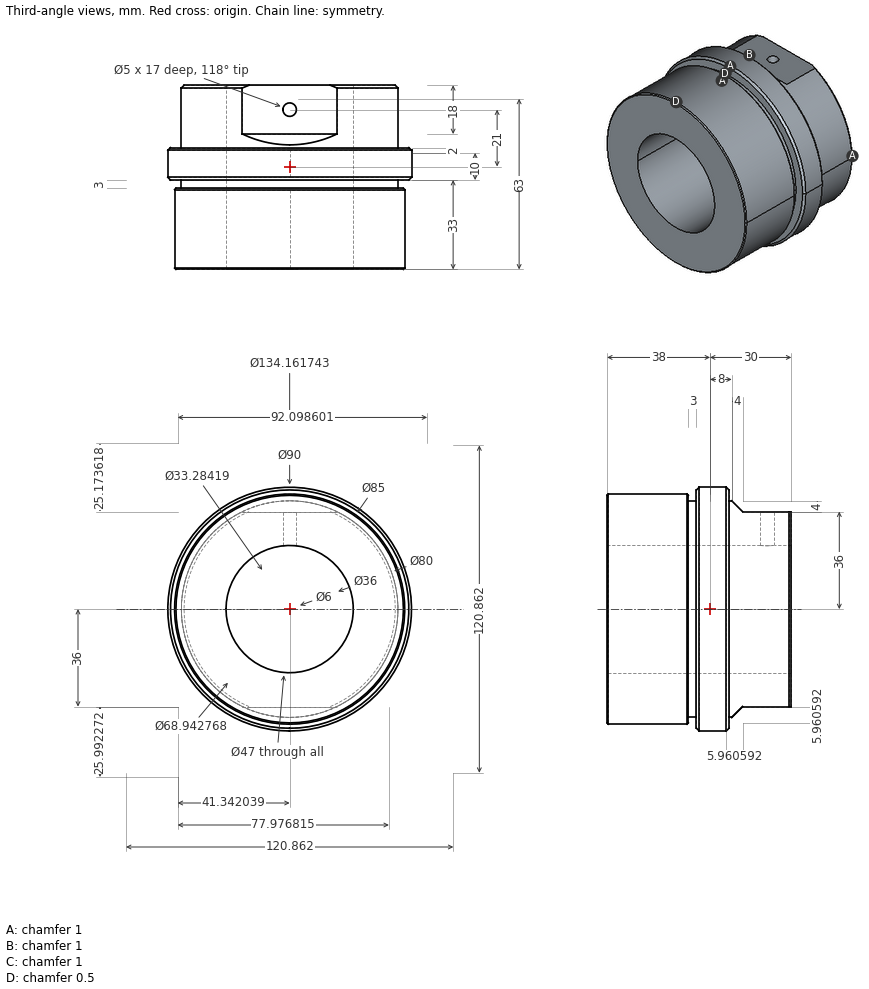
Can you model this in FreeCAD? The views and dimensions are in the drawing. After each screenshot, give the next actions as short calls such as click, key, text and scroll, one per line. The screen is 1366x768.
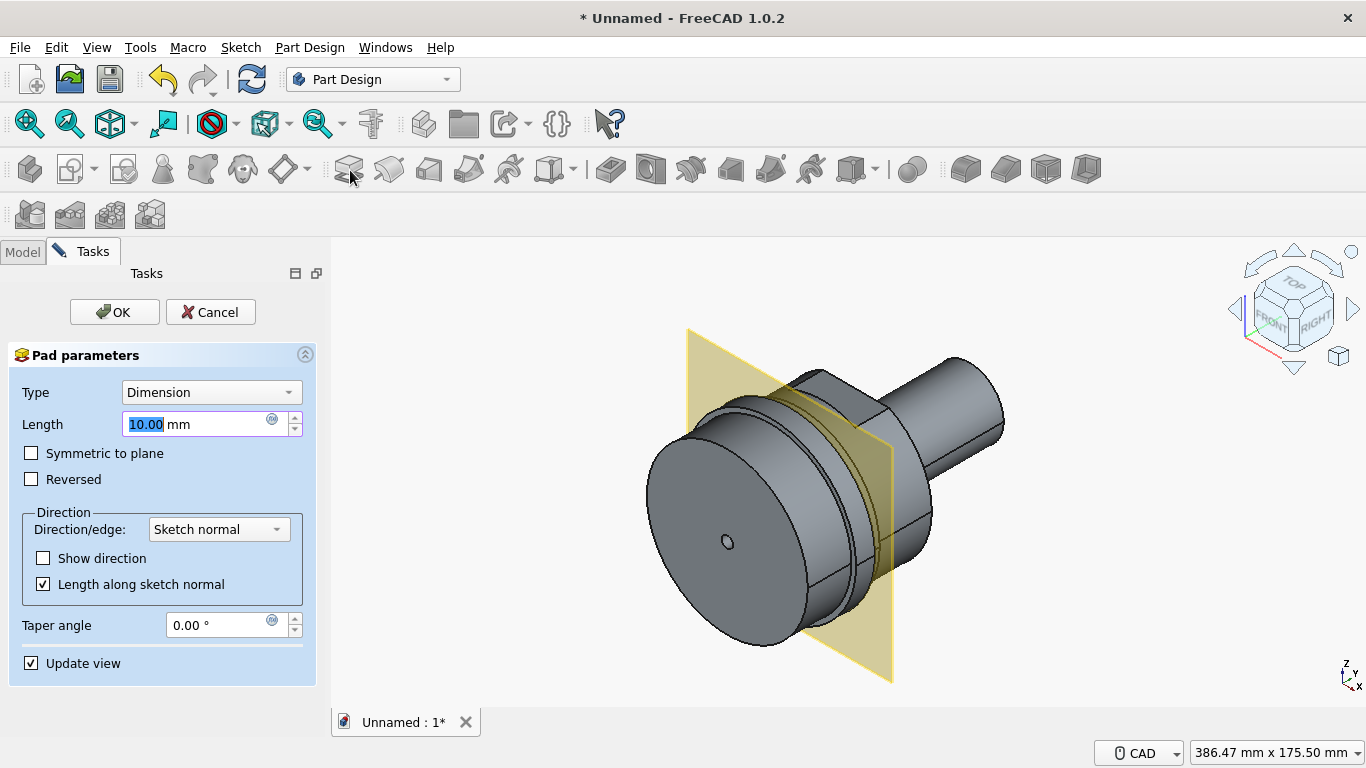
text(10)
key(Tab)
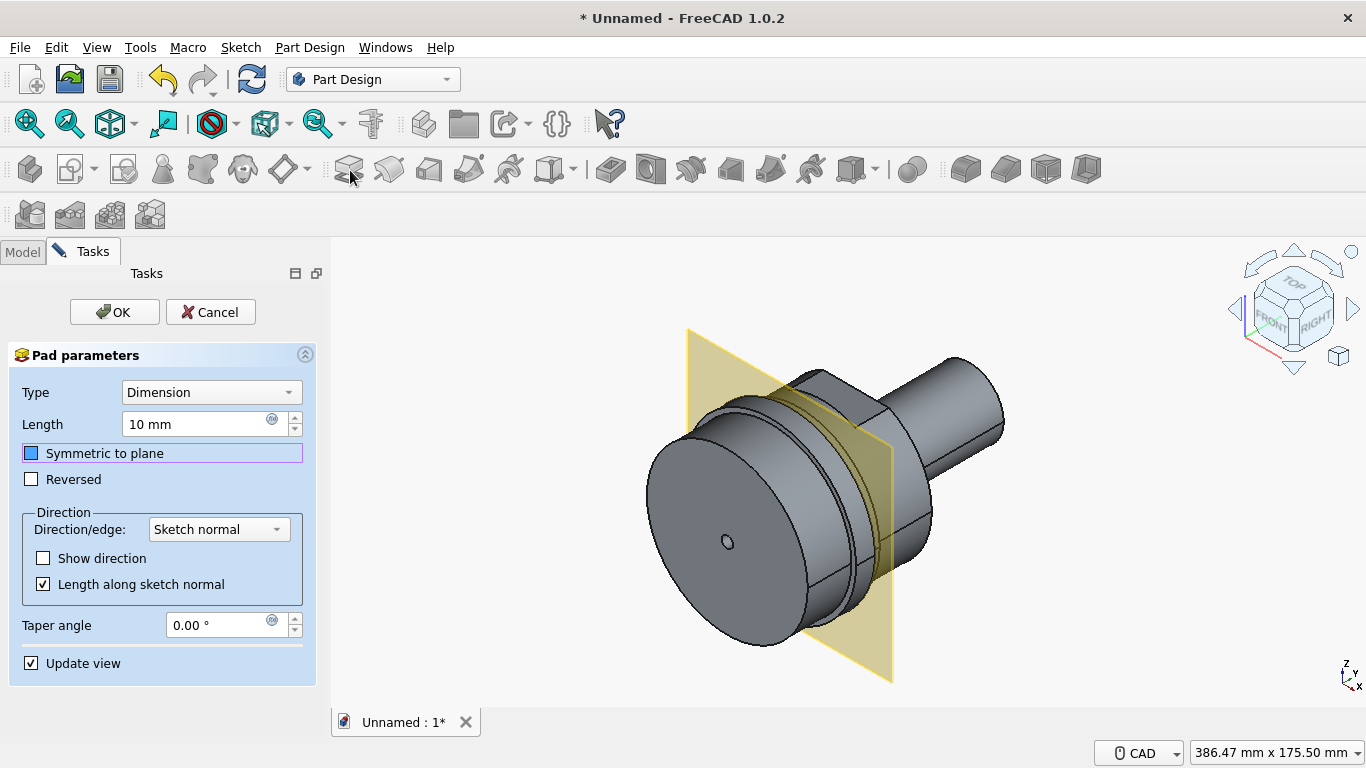
click(30, 479)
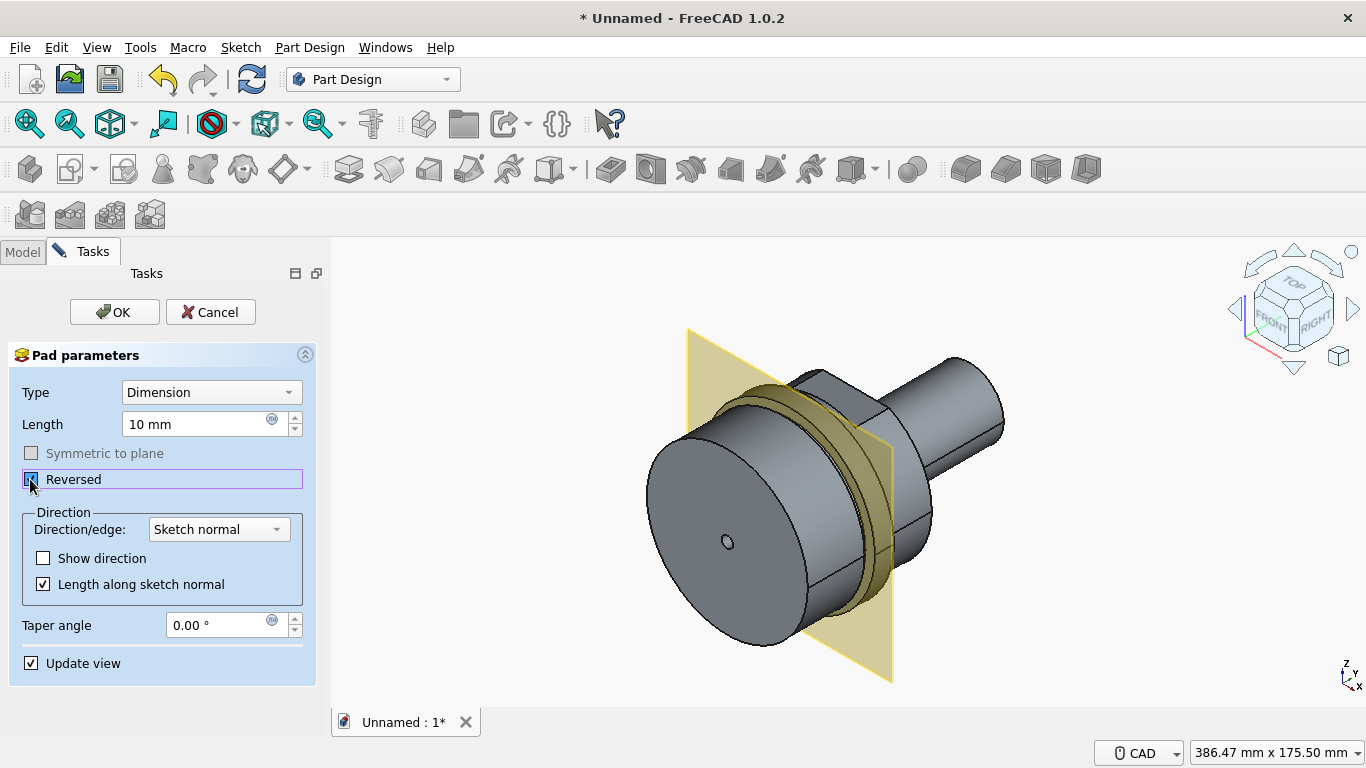
click(115, 312)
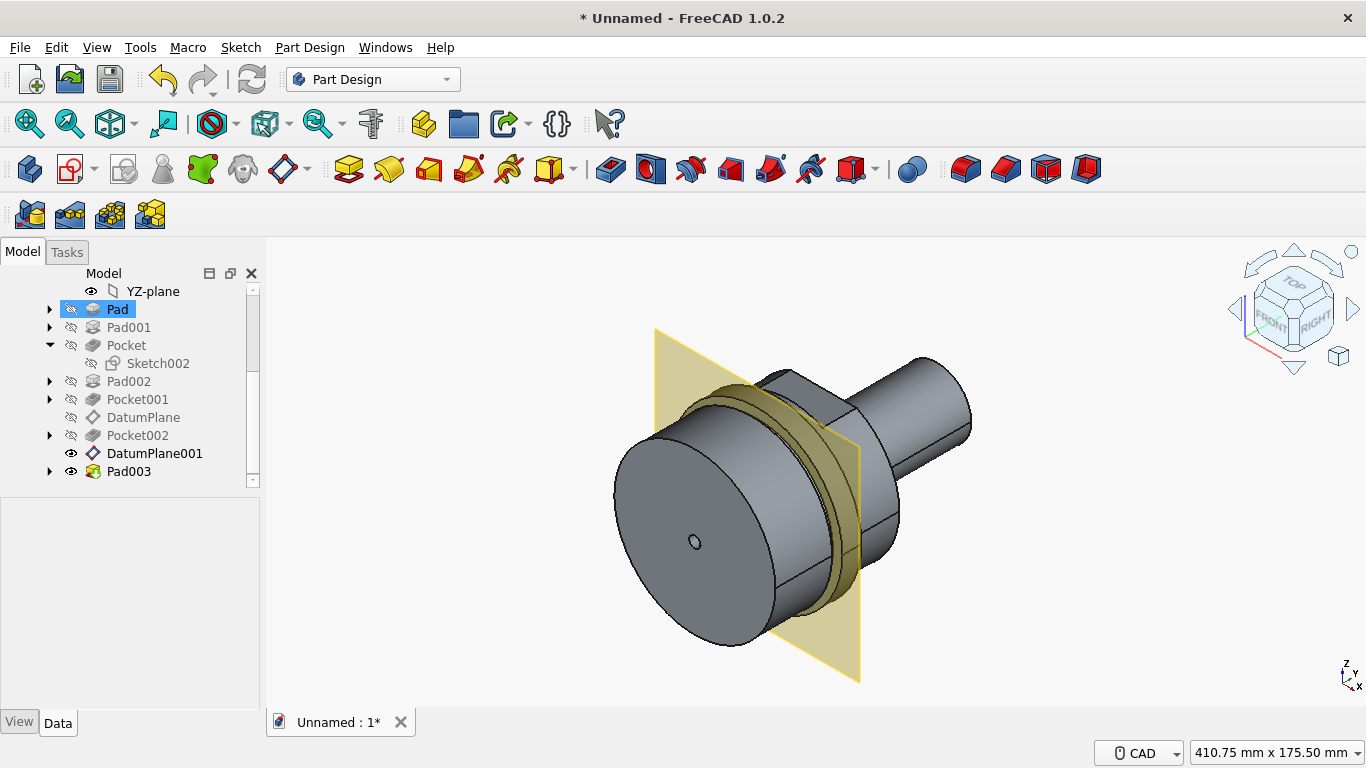
click(116, 453)
key(space)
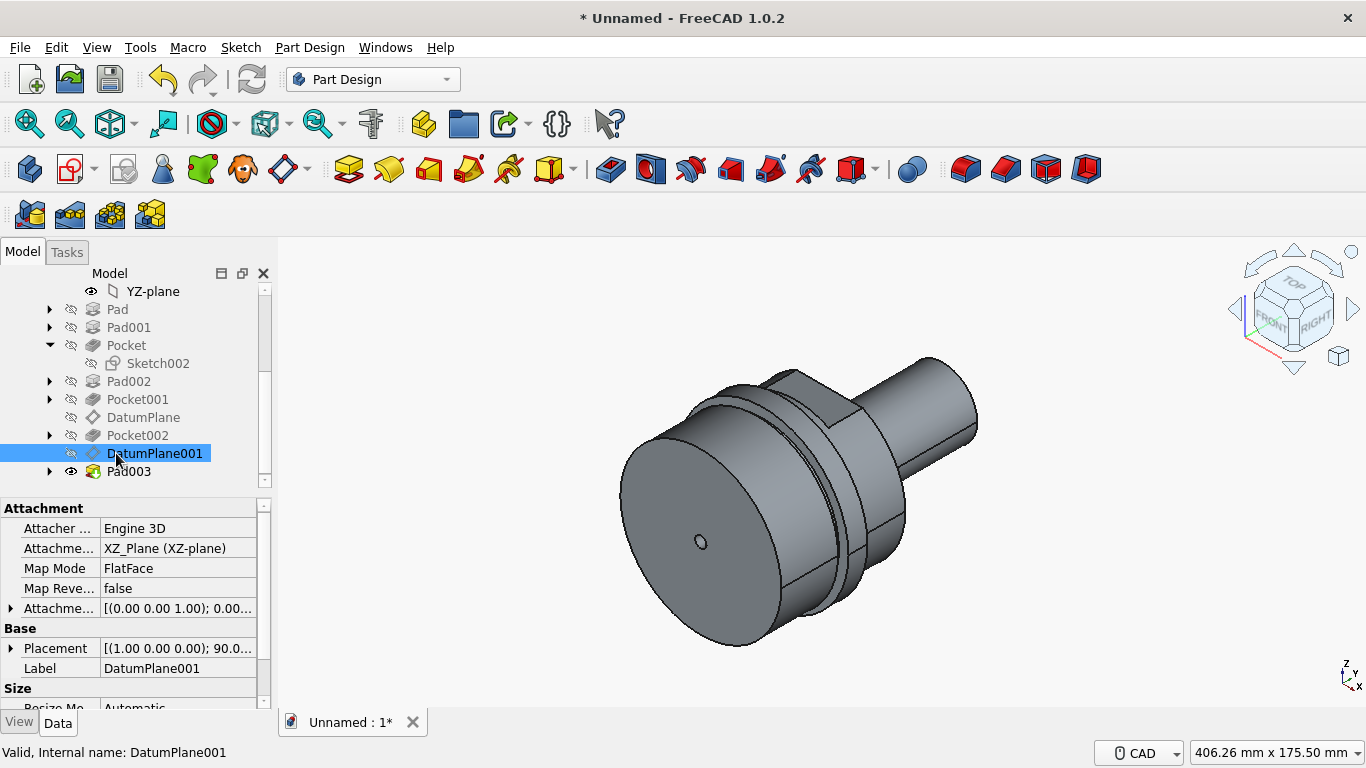
click(676, 438)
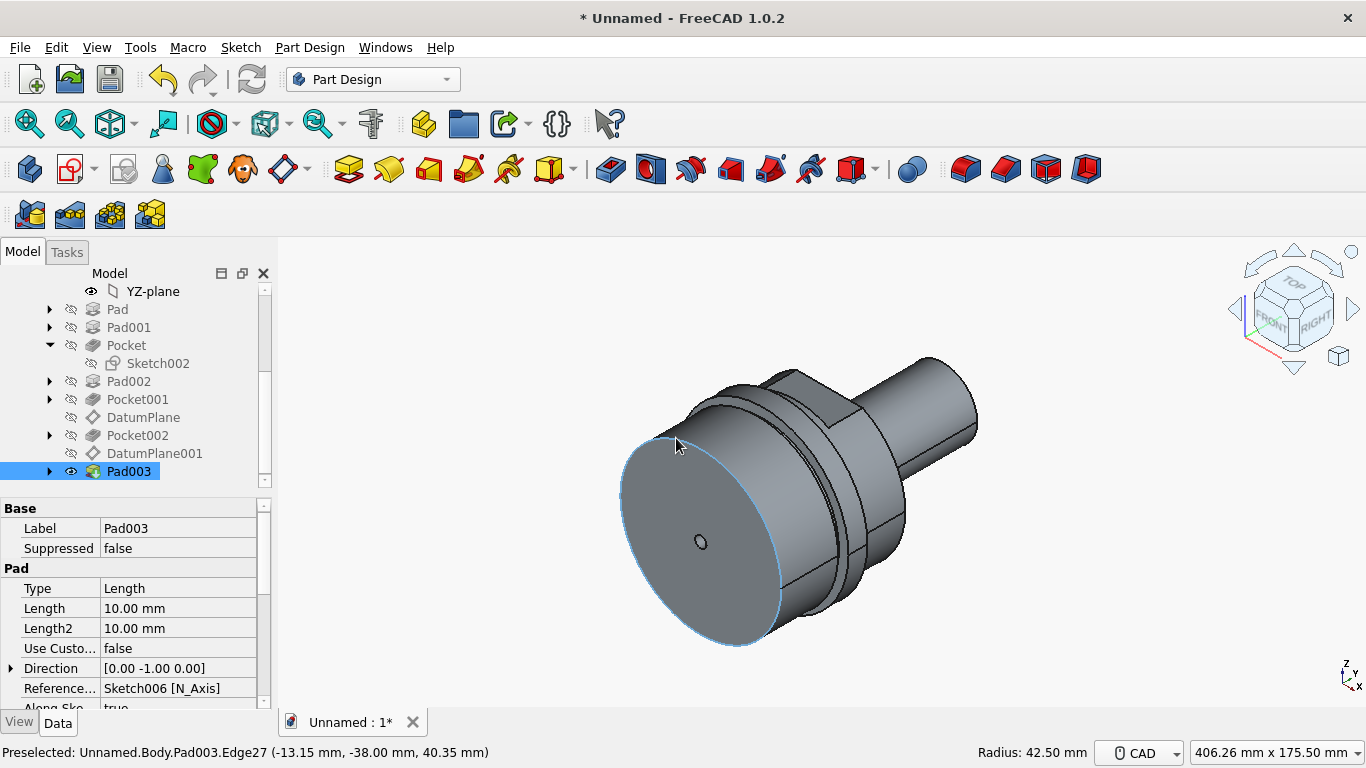
click(737, 396, ctrl)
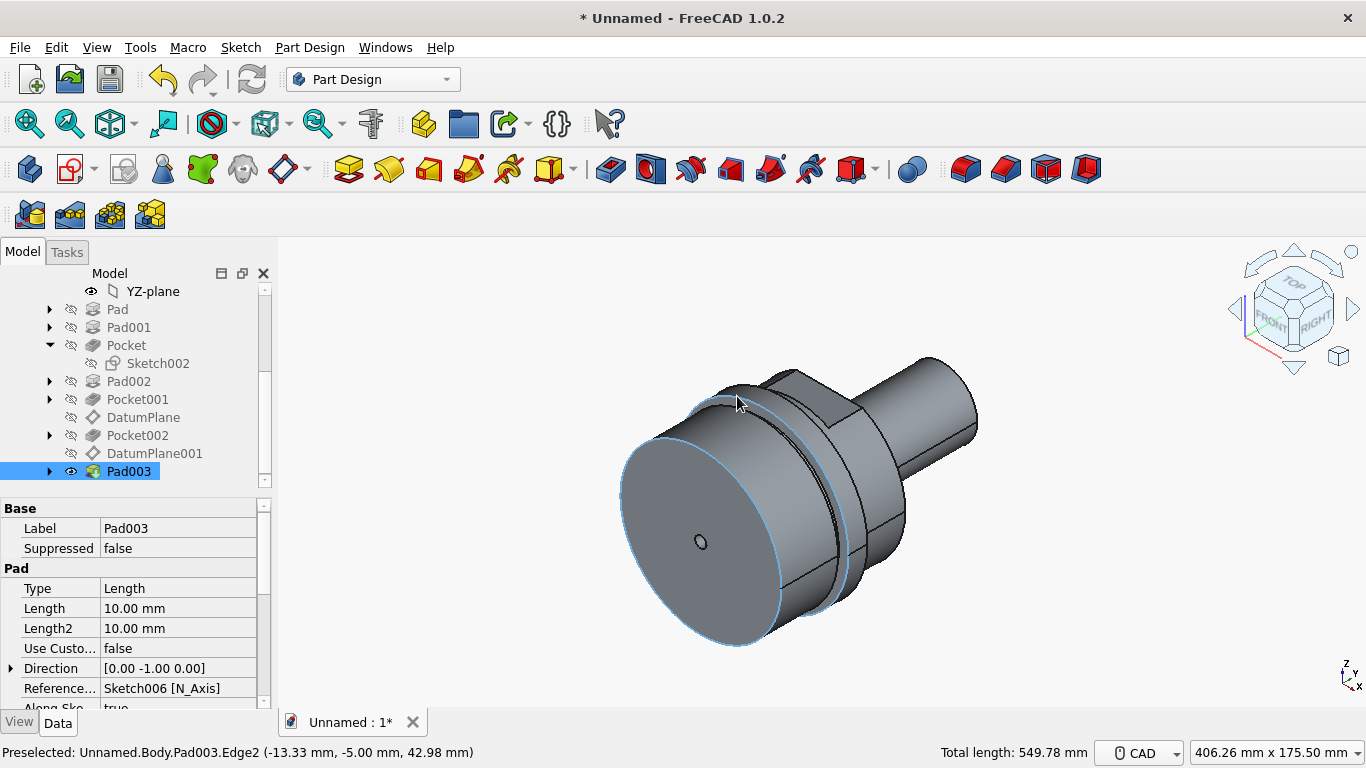
key(2)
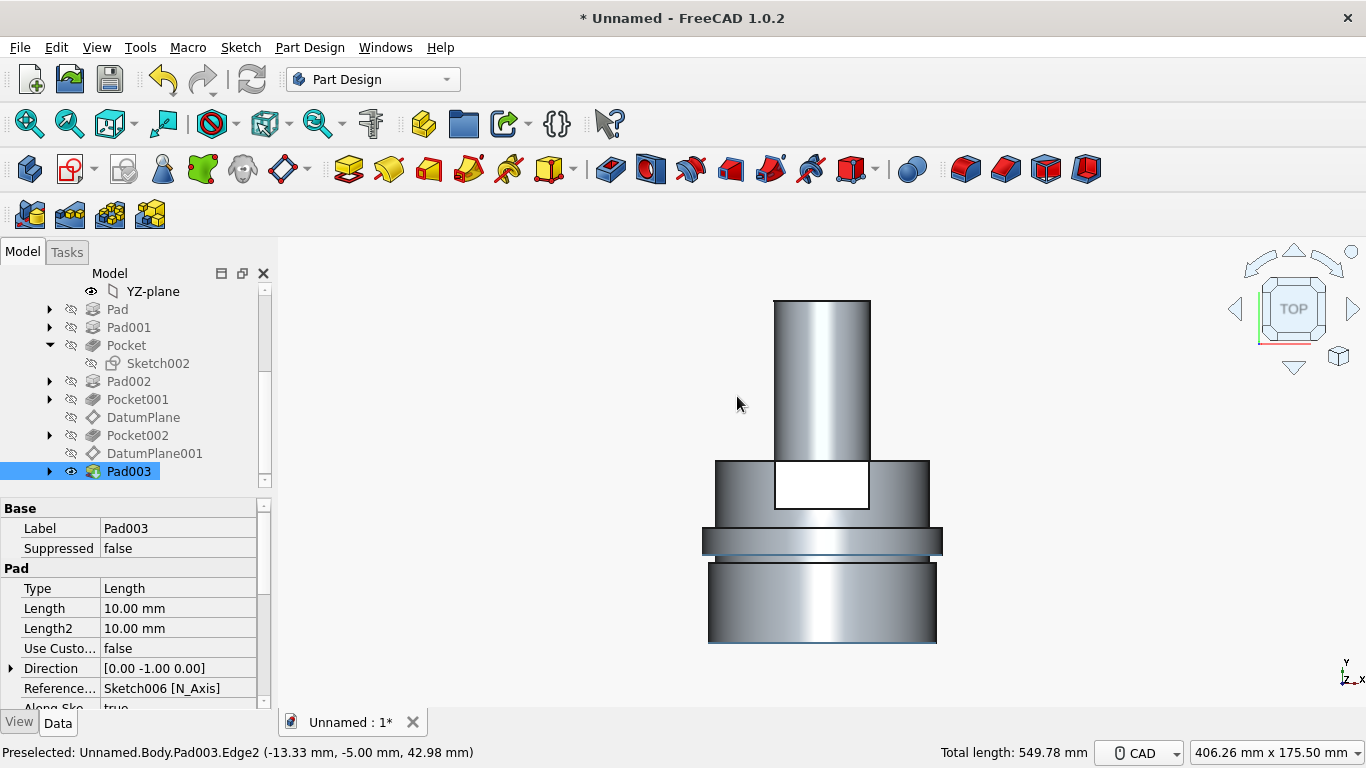
click(783, 300, ctrl)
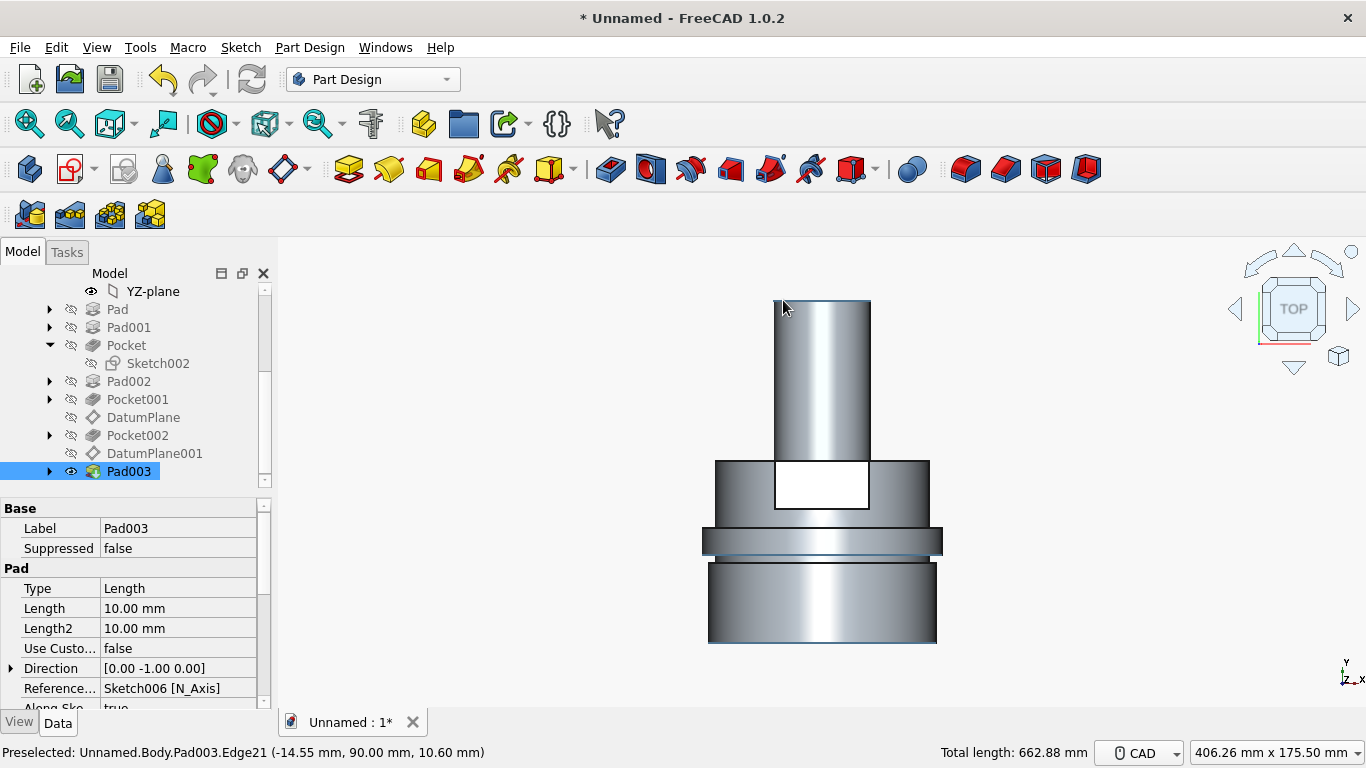
click(738, 460, ctrl)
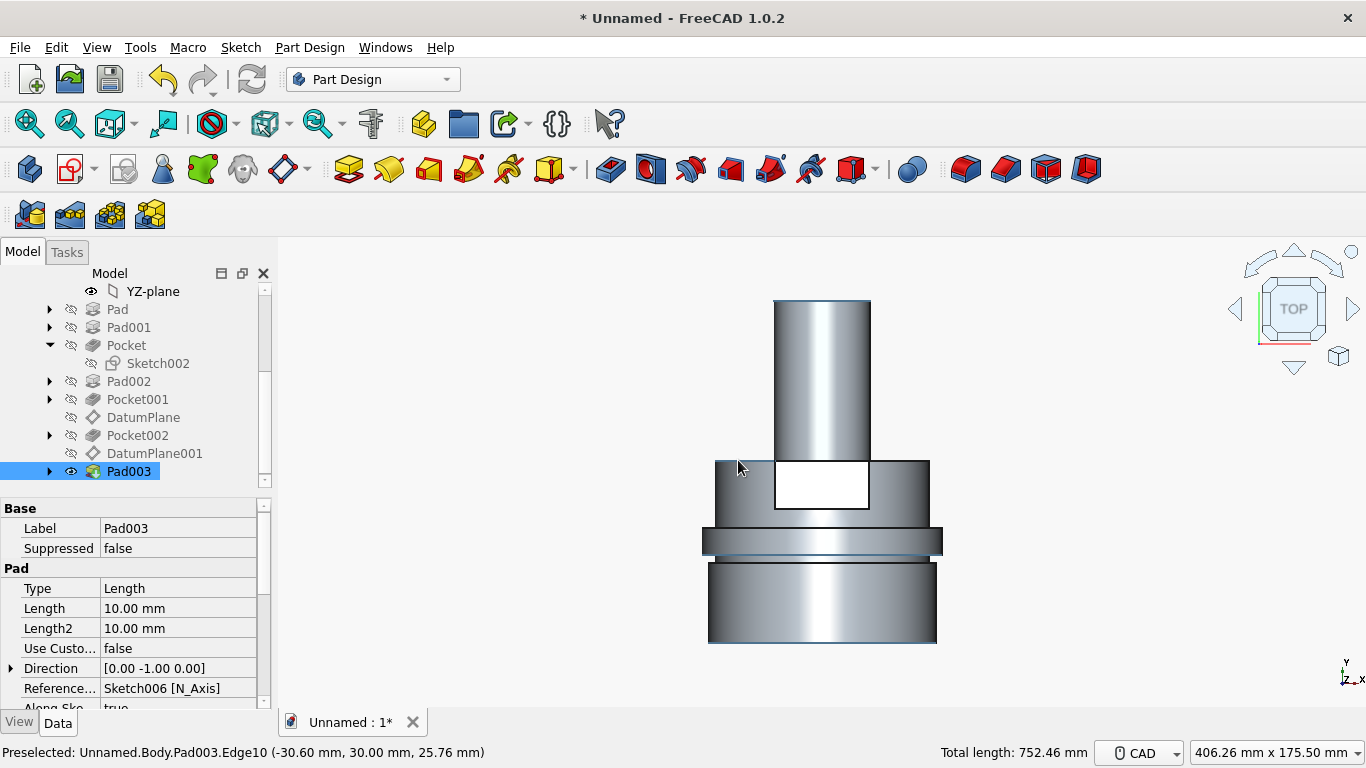
key(0)